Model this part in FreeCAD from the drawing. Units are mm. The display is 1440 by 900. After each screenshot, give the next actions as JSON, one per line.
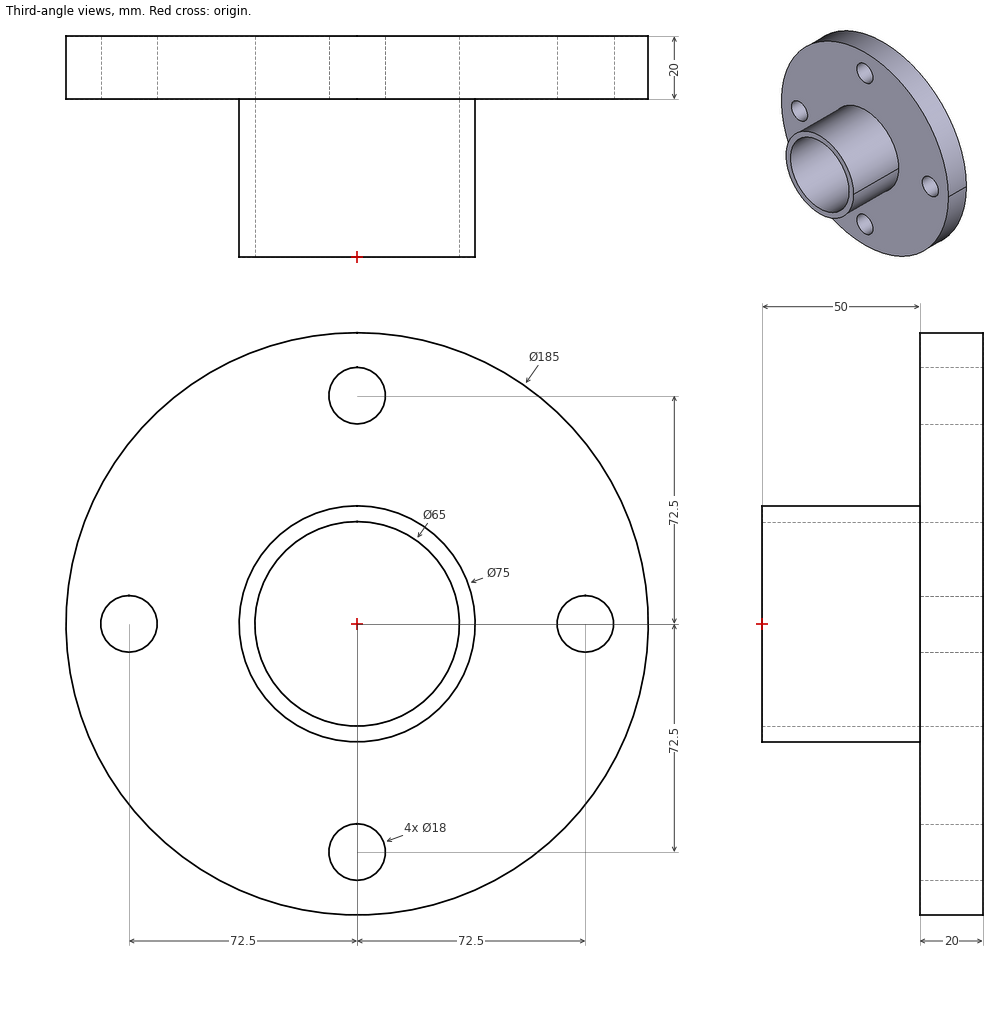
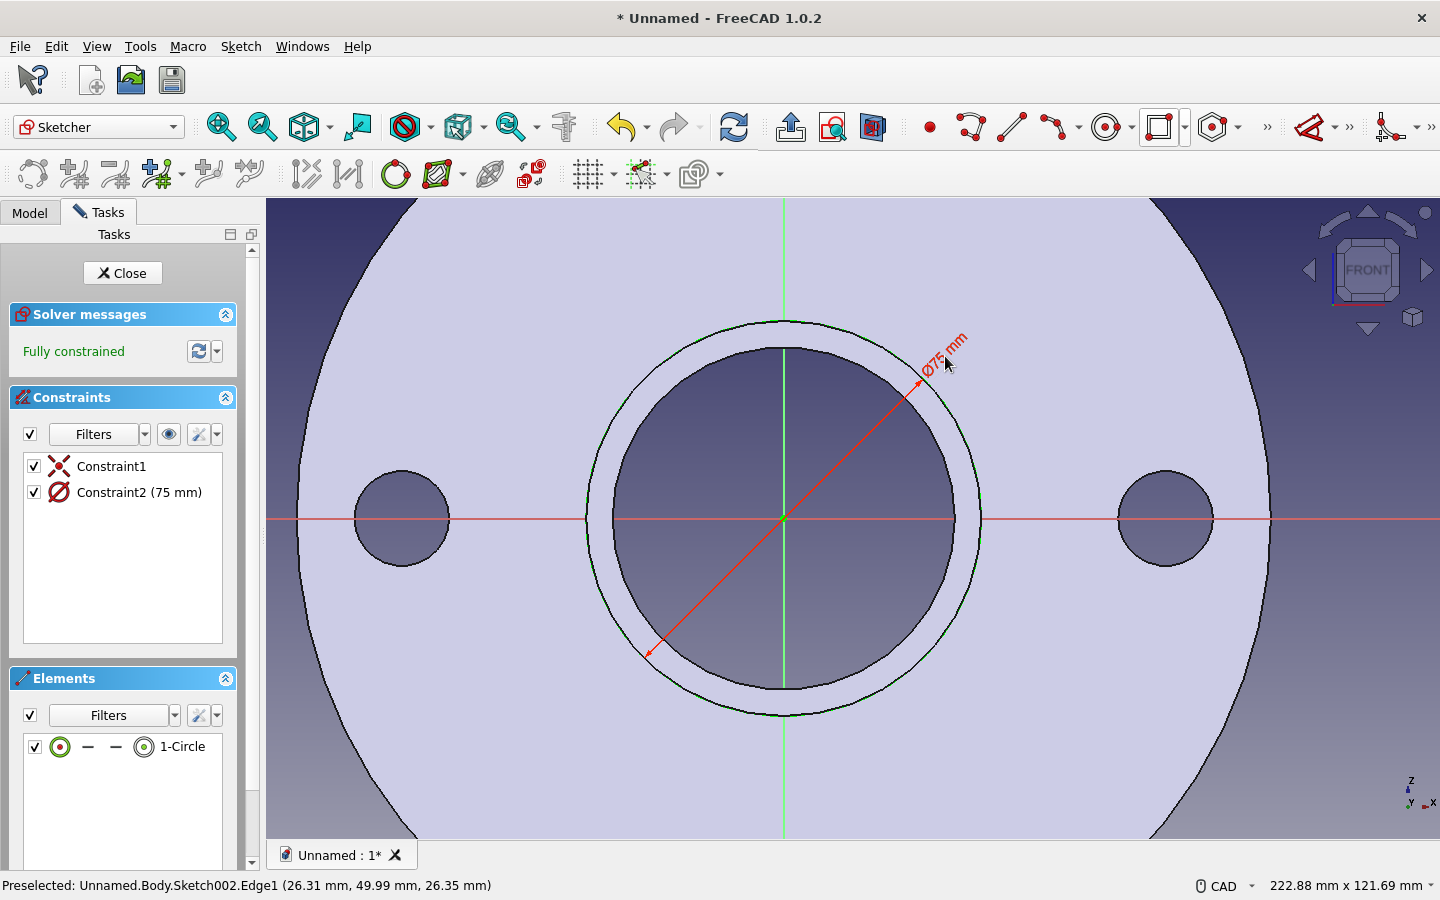
{"action": "left_click", "coordinate": [123, 273]}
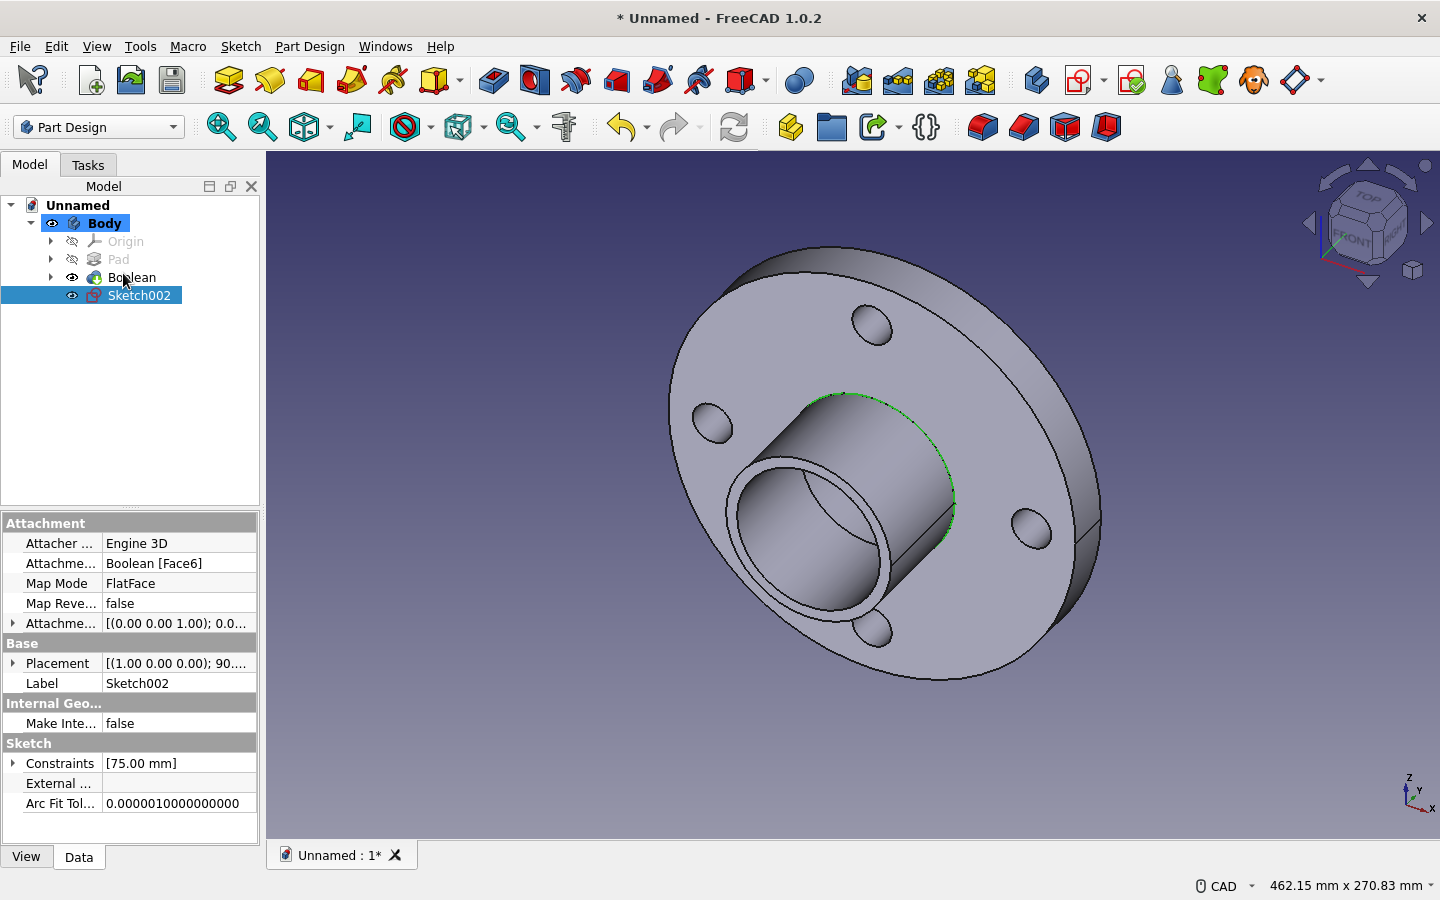
{"action": "left_click", "coordinate": [229, 80]}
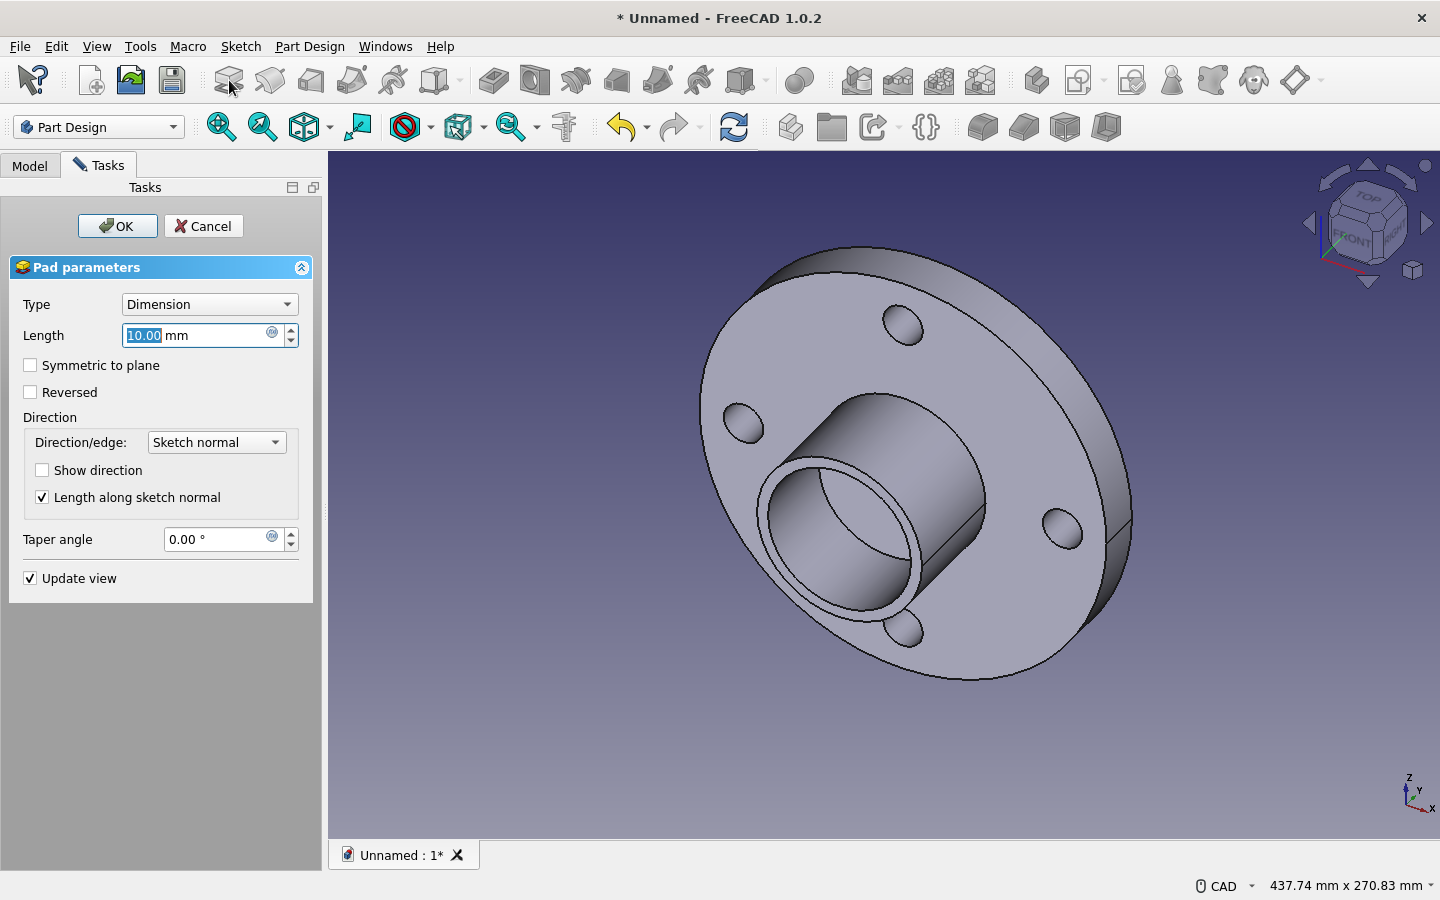
{"action": "type", "text": "20"}
{"action": "key", "text": "Tab"}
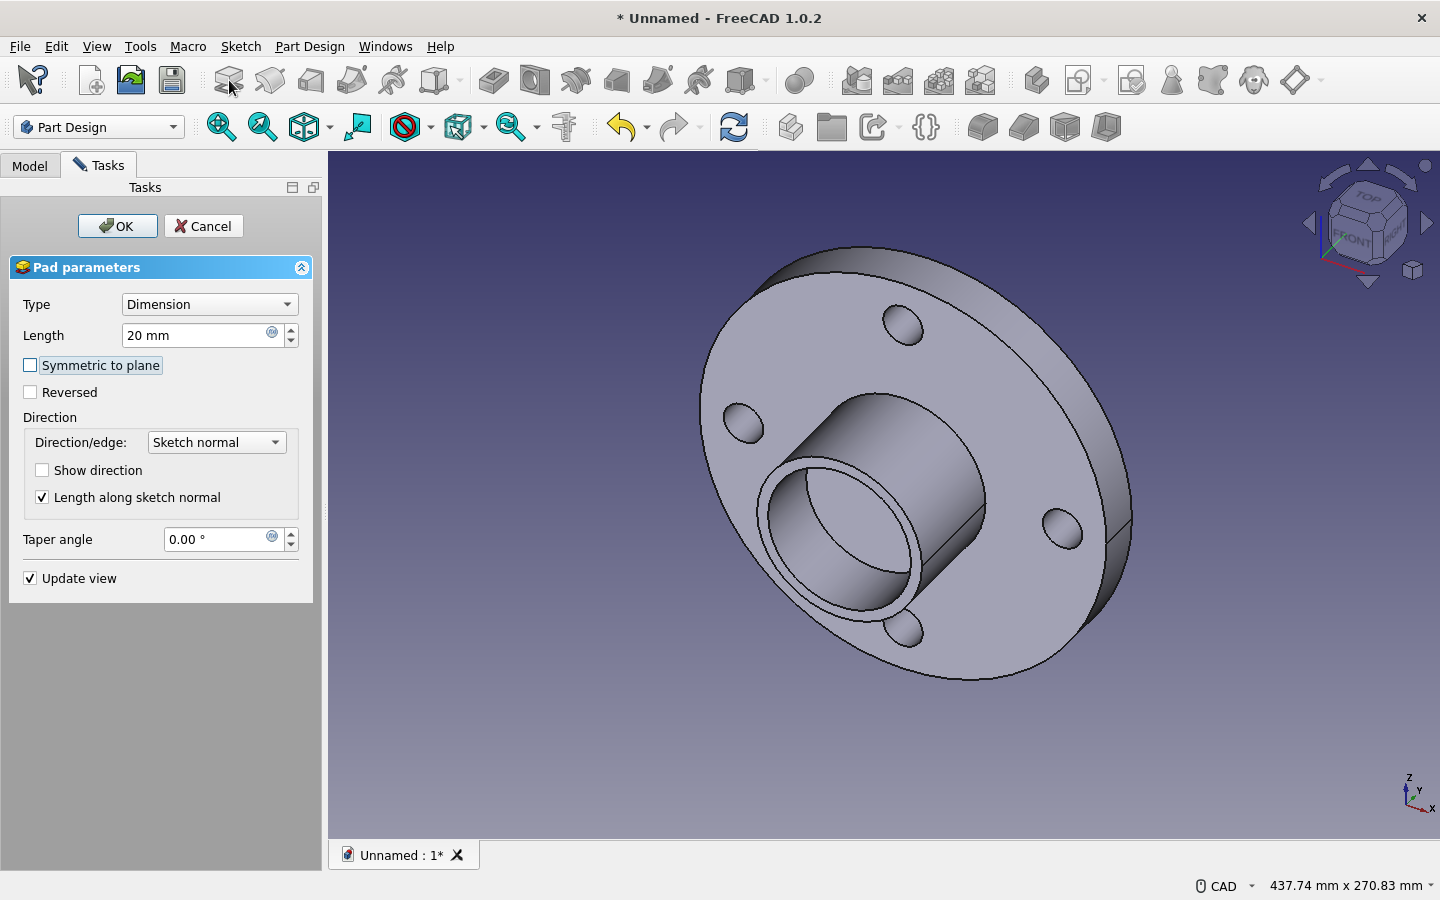
{"action": "left_click", "coordinate": [31, 392]}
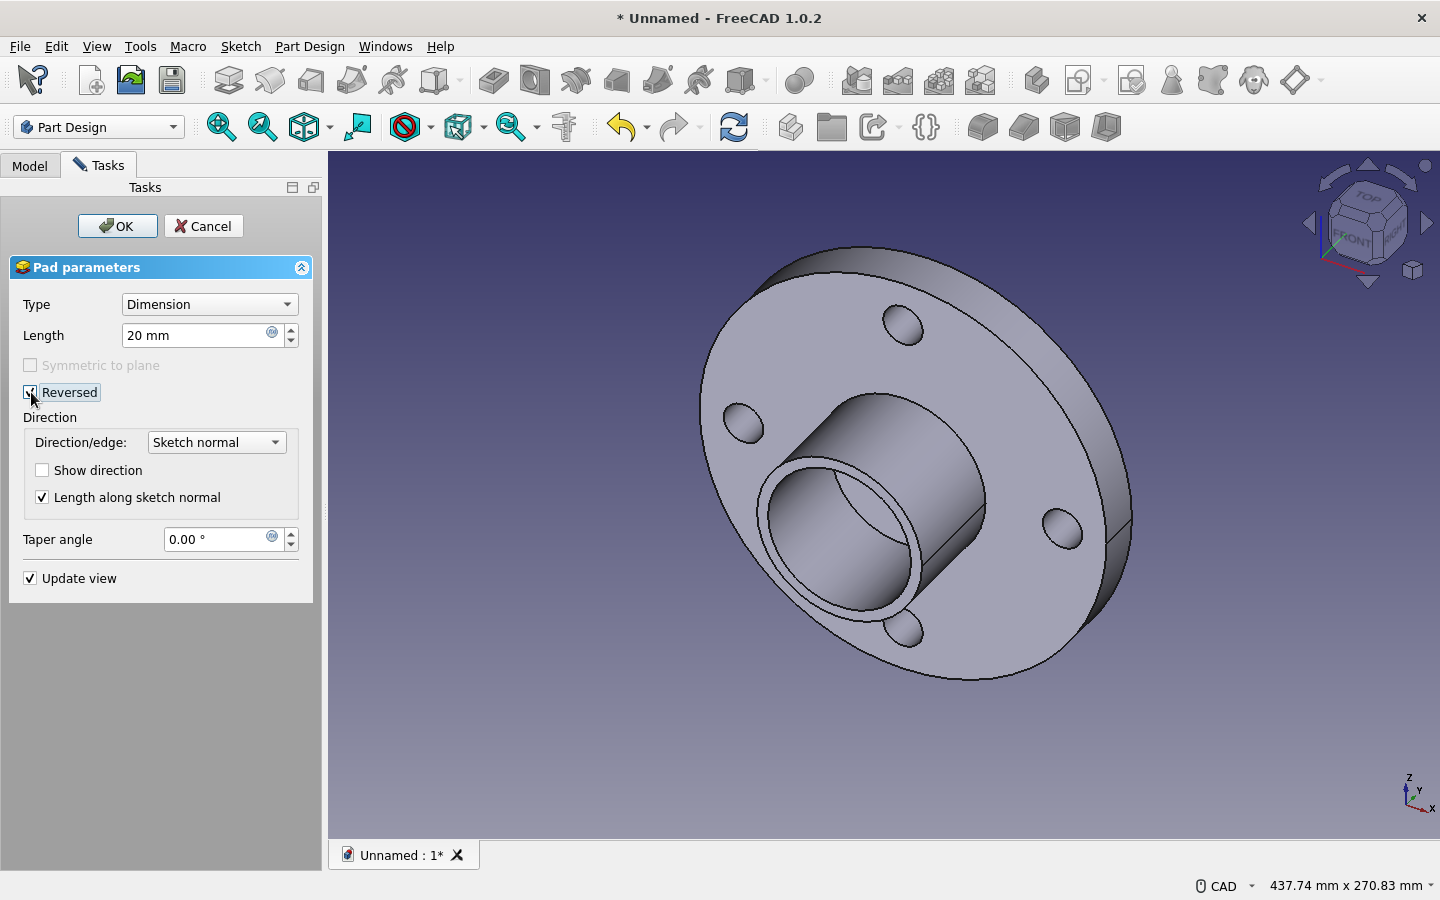
{"action": "left_click", "coordinate": [118, 226]}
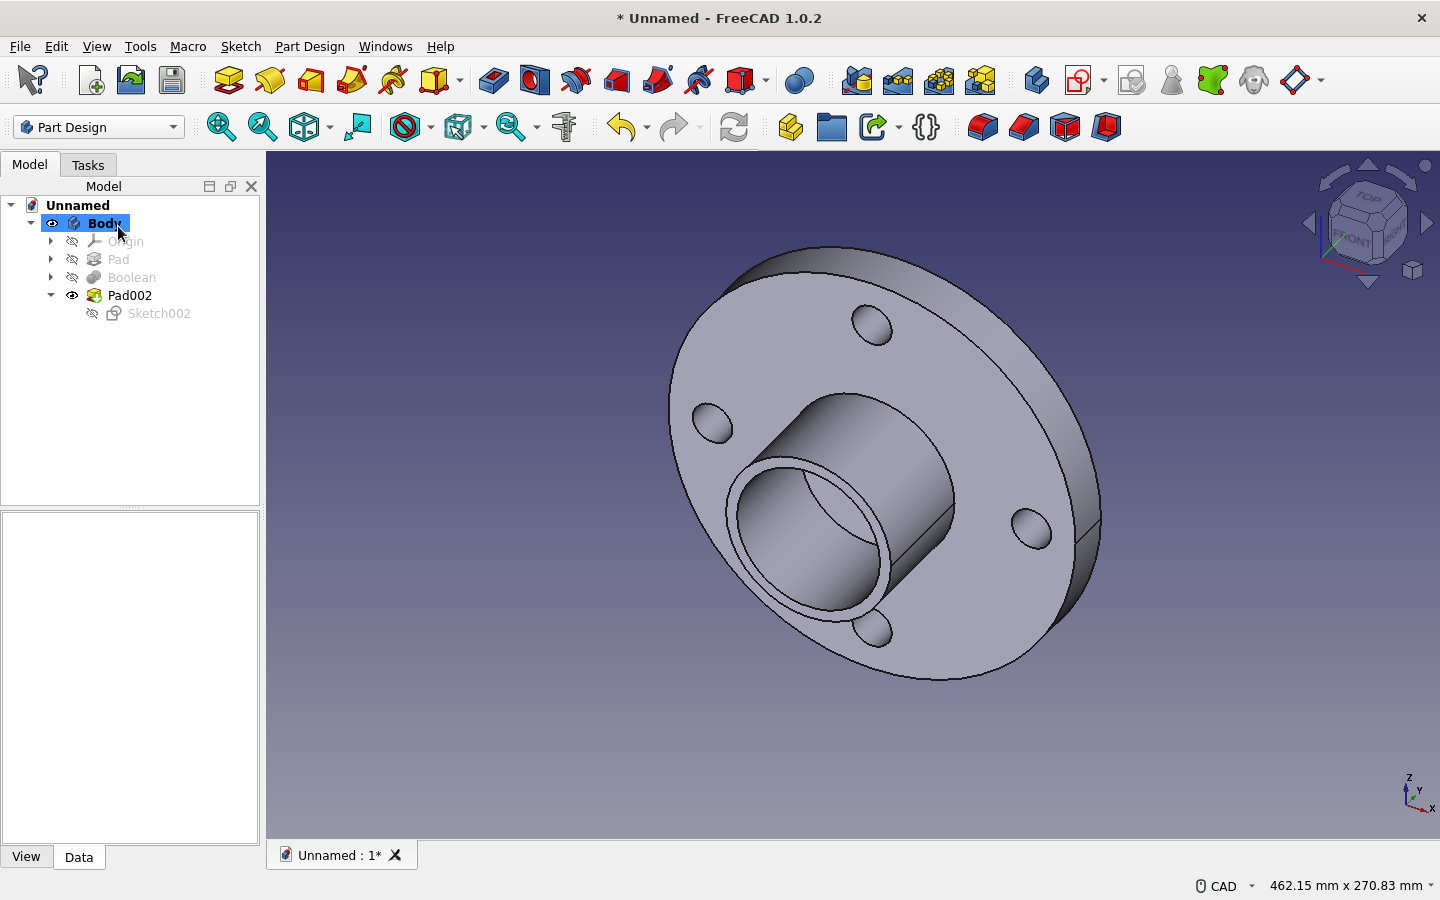
{"action": "left_click", "coordinate": [814, 346]}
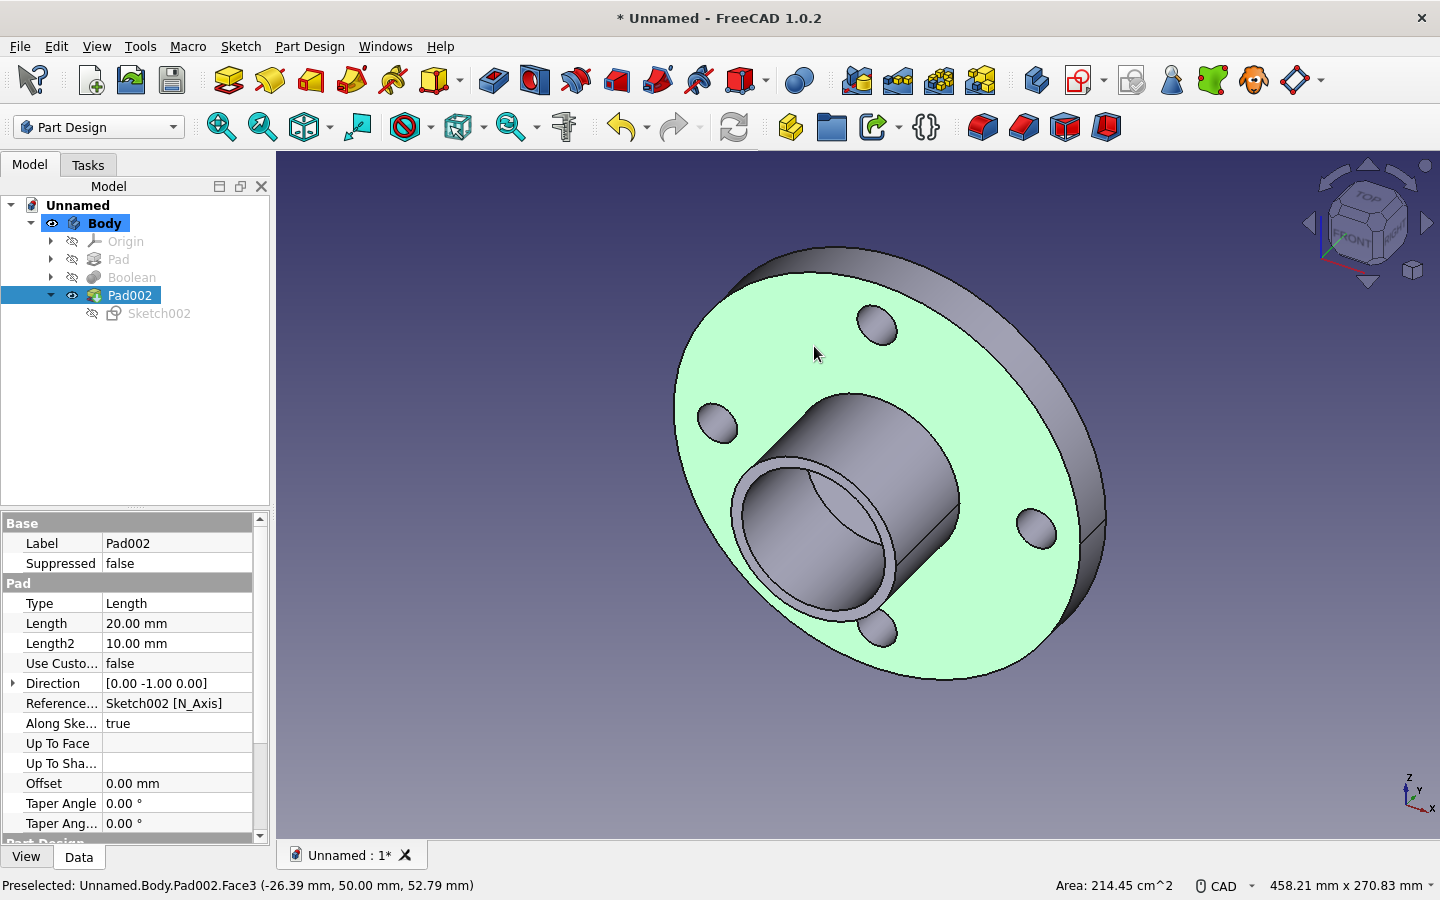
{"action": "left_click", "coordinate": [1078, 80]}